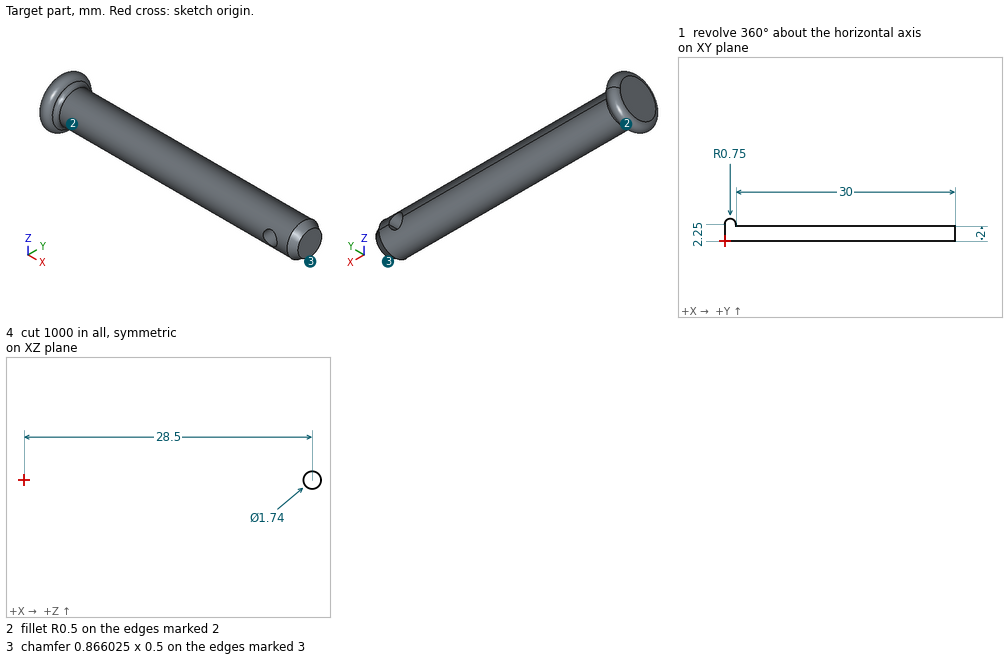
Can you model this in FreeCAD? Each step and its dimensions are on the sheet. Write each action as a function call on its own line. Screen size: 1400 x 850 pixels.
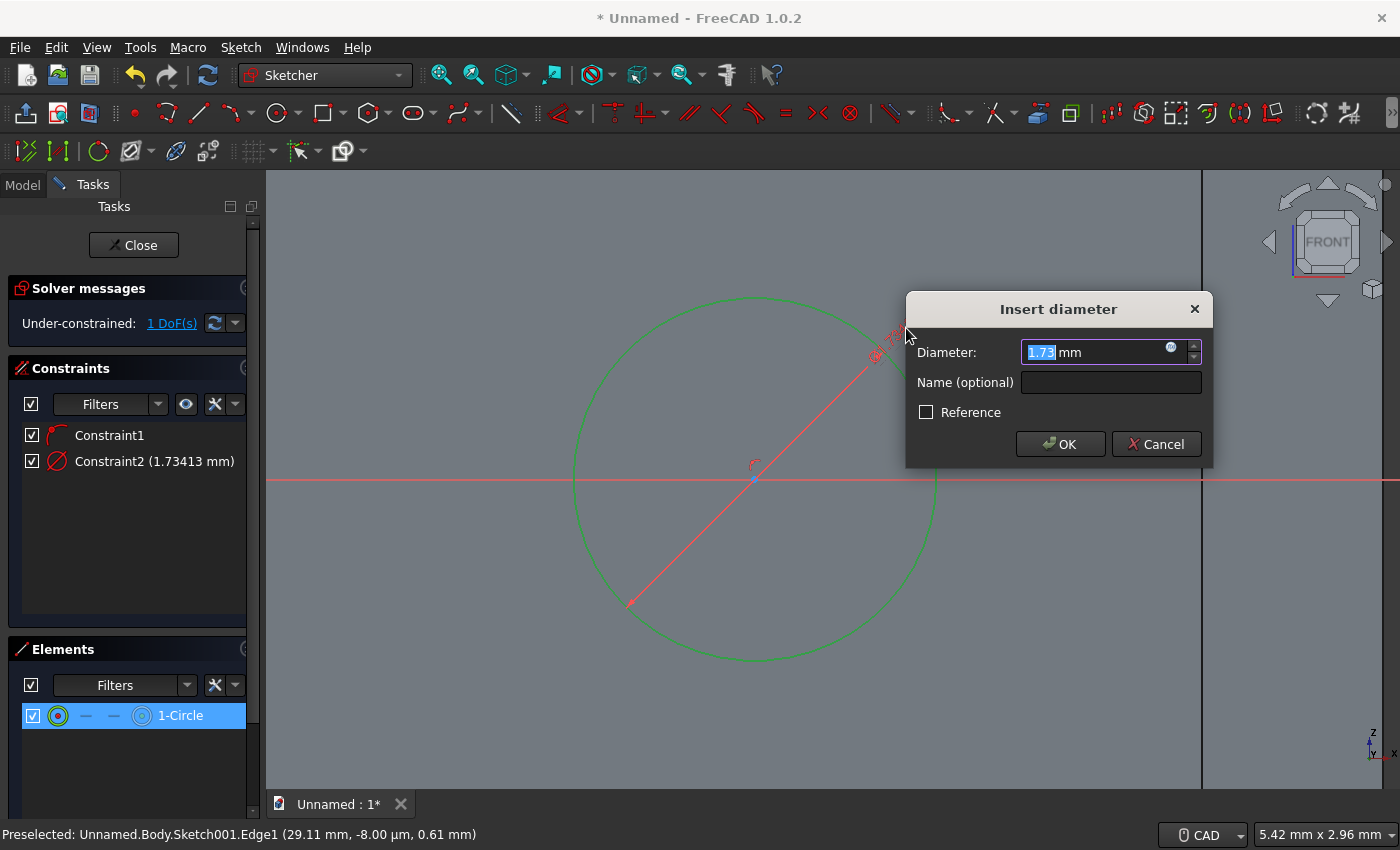
text(1.74)
key(Return)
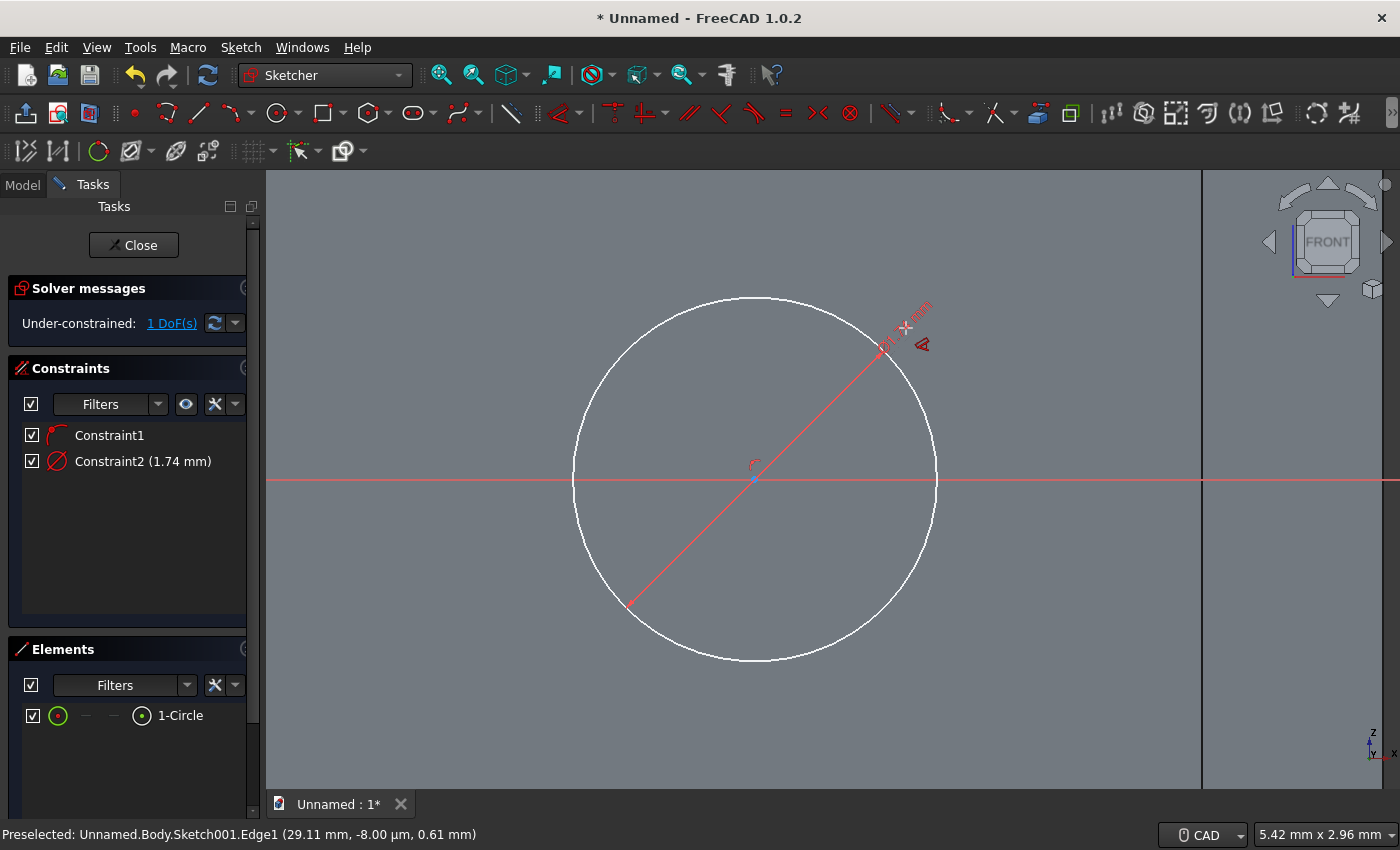
click(755, 479)
click(524, 513)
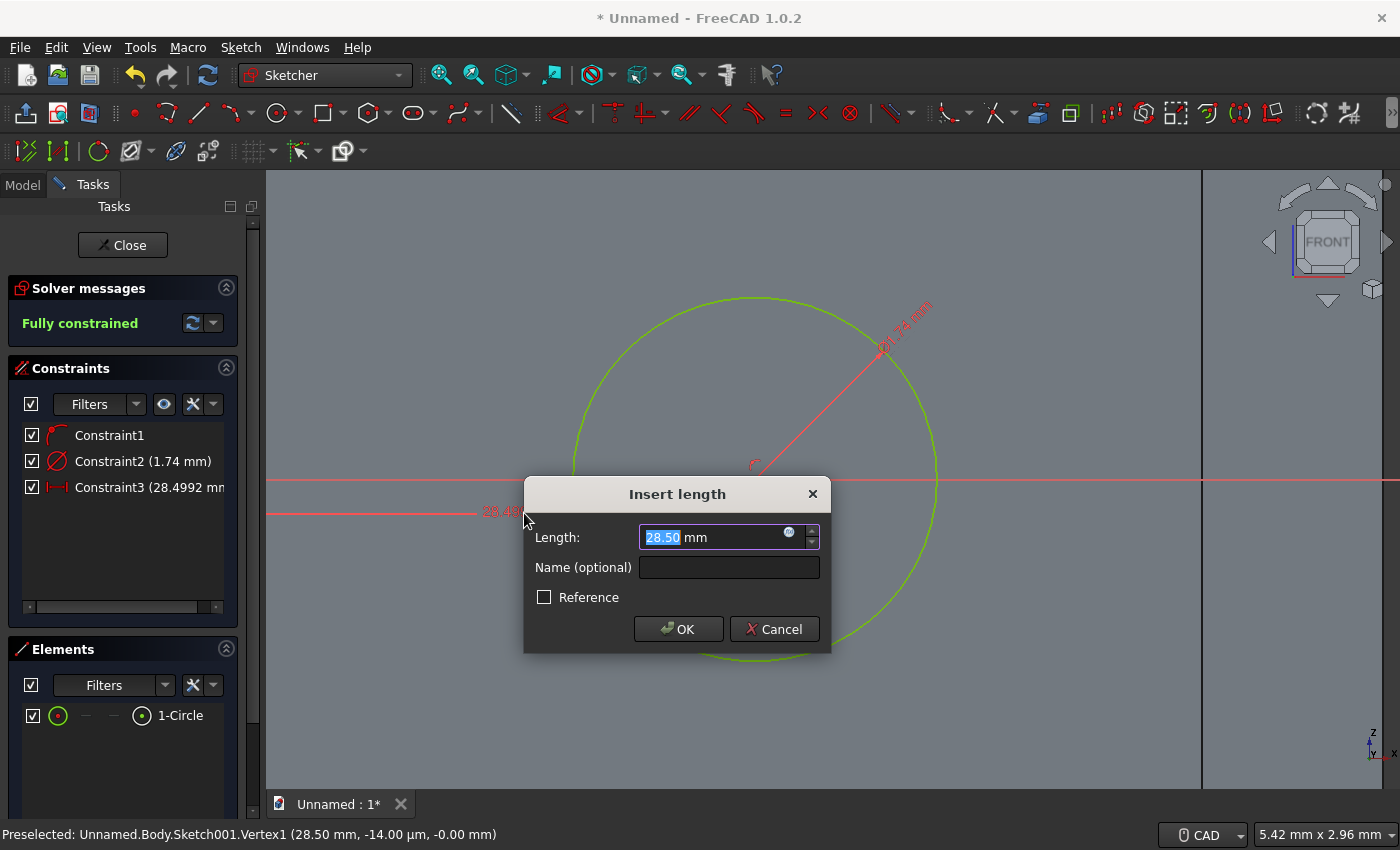
text(28.5)
key(Return)
key(Escape)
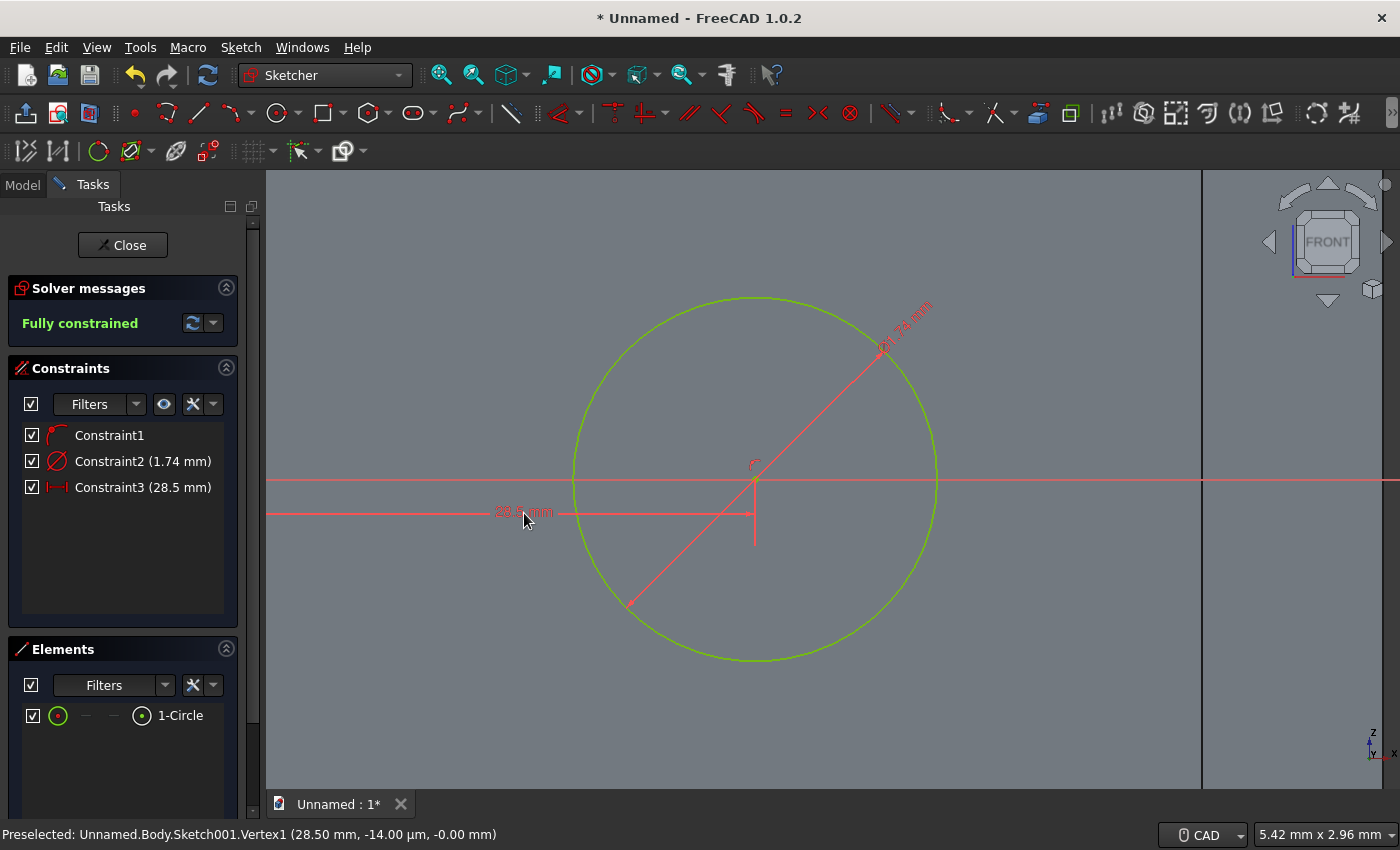
click(123, 245)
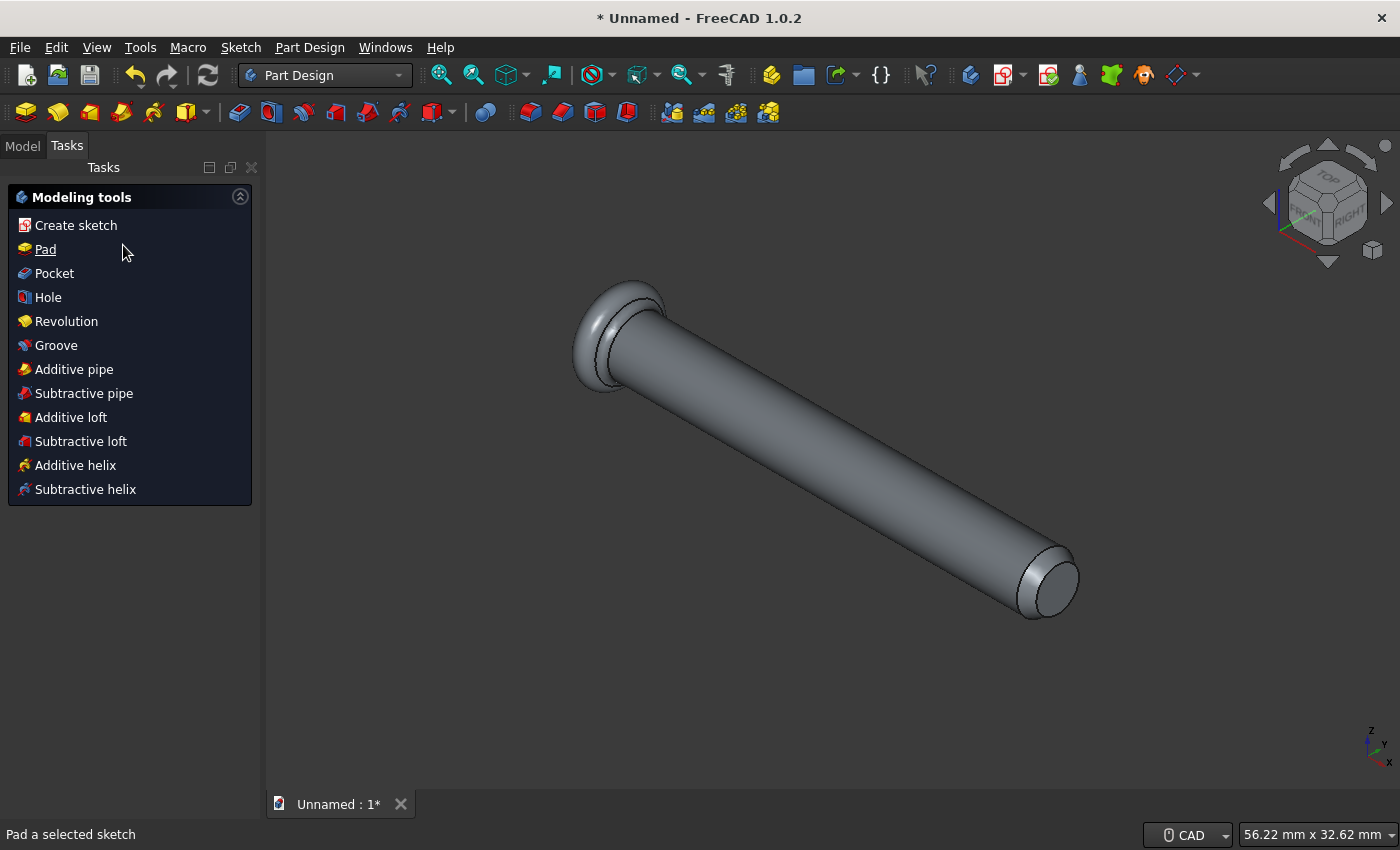
click(240, 112)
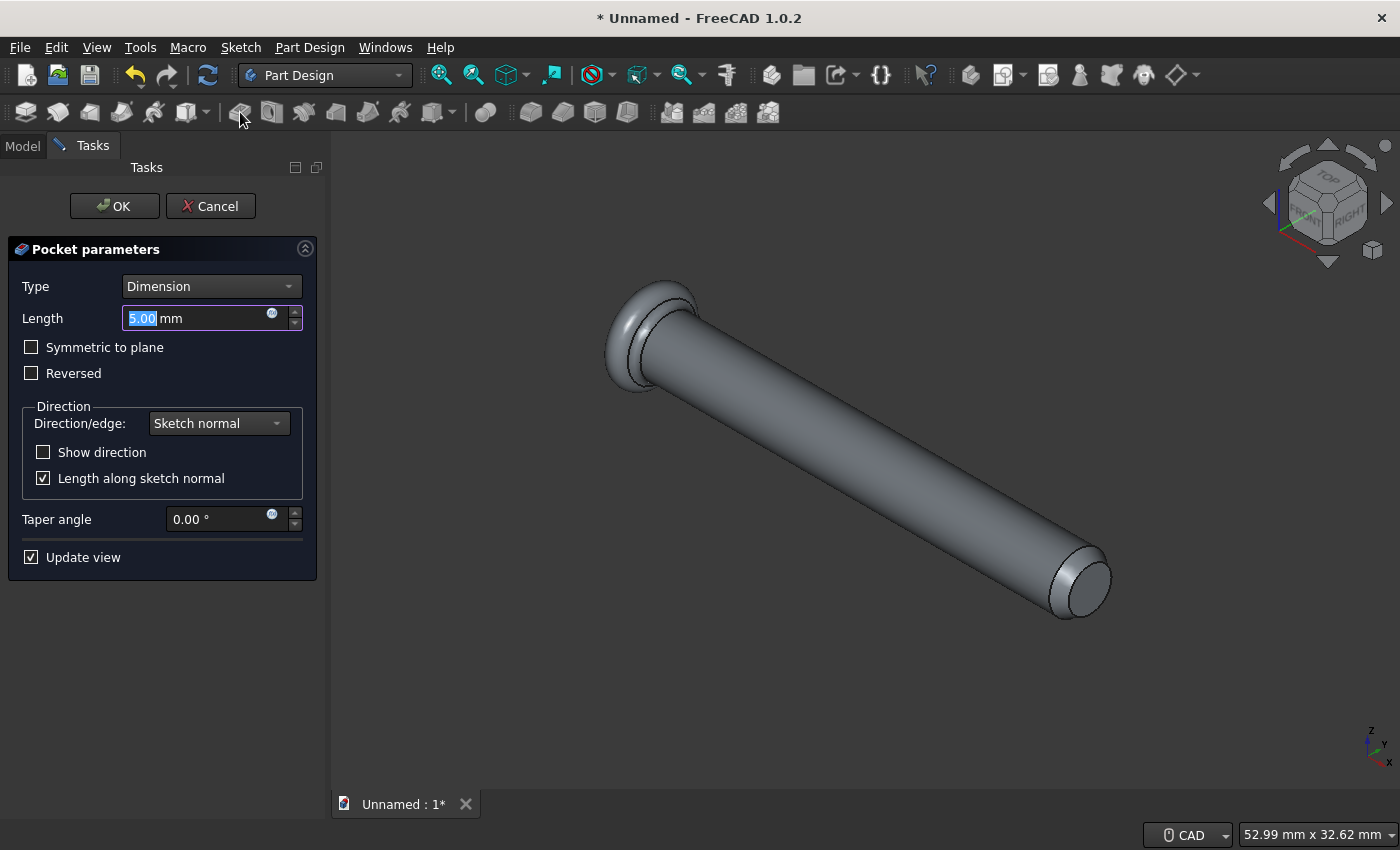
text(1000)
key(Tab)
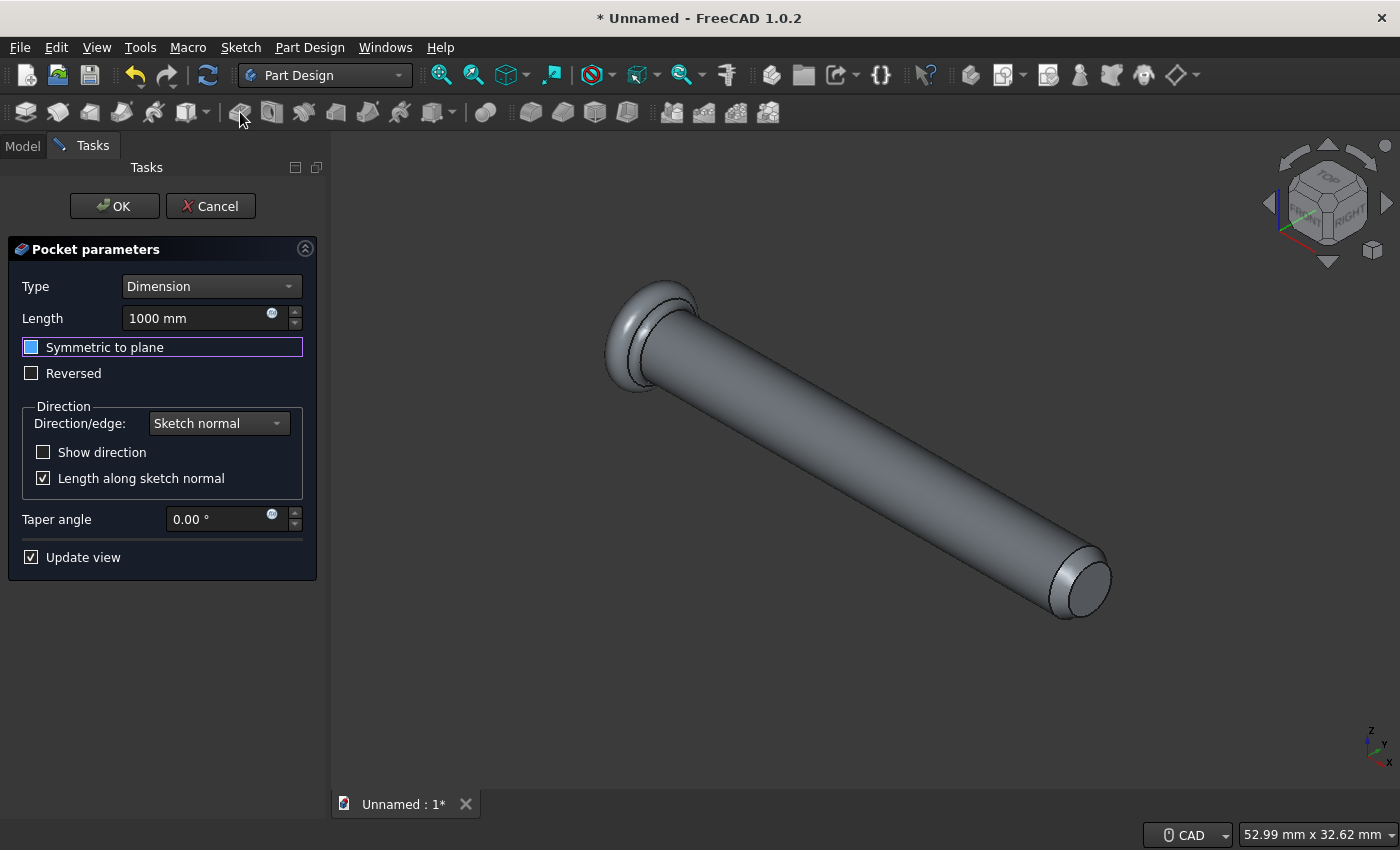
click(30, 347)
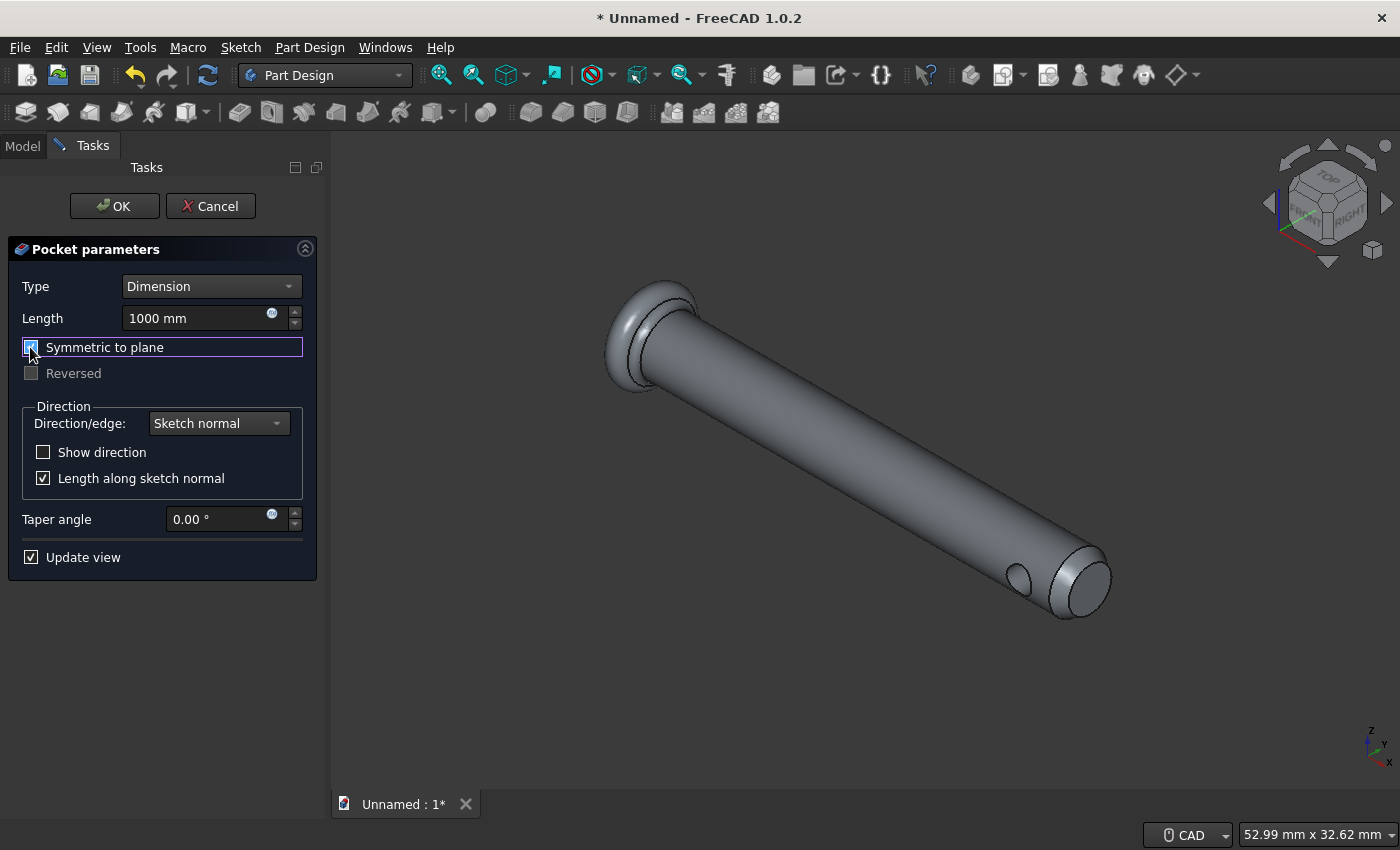
click(115, 206)